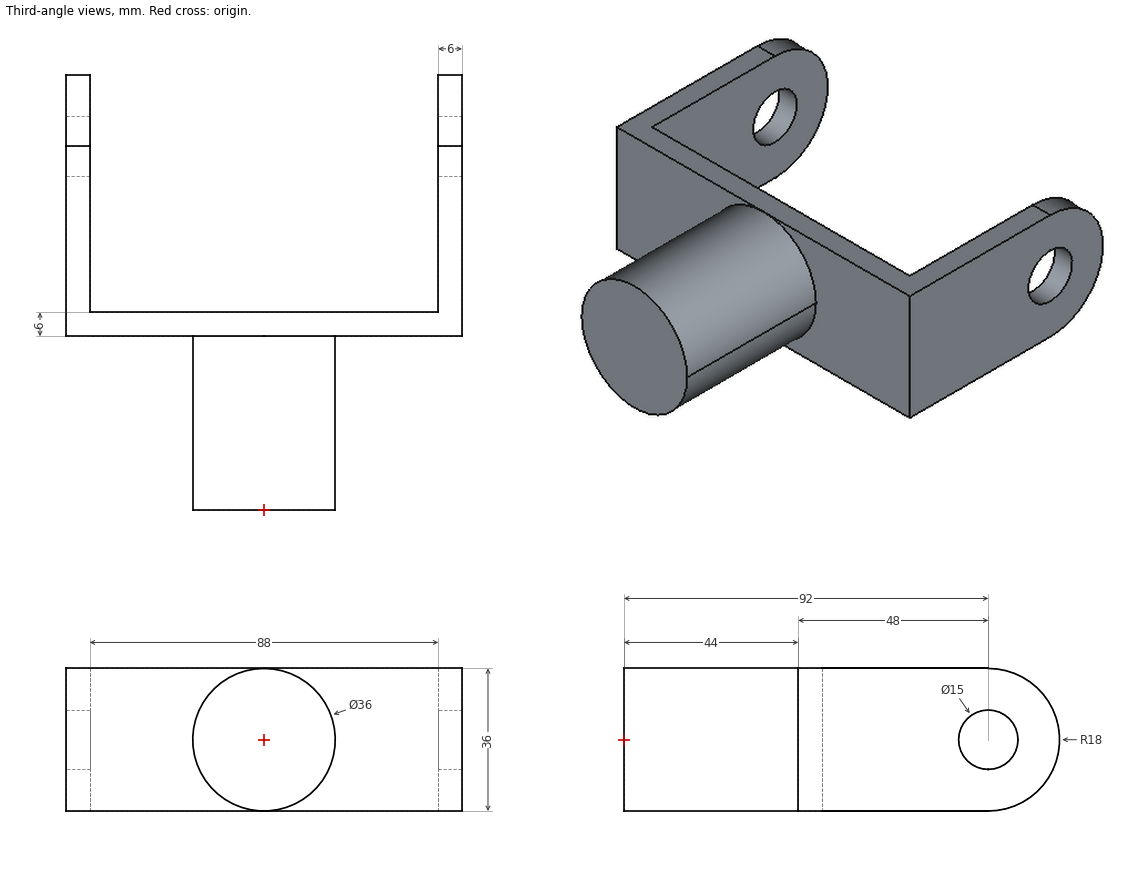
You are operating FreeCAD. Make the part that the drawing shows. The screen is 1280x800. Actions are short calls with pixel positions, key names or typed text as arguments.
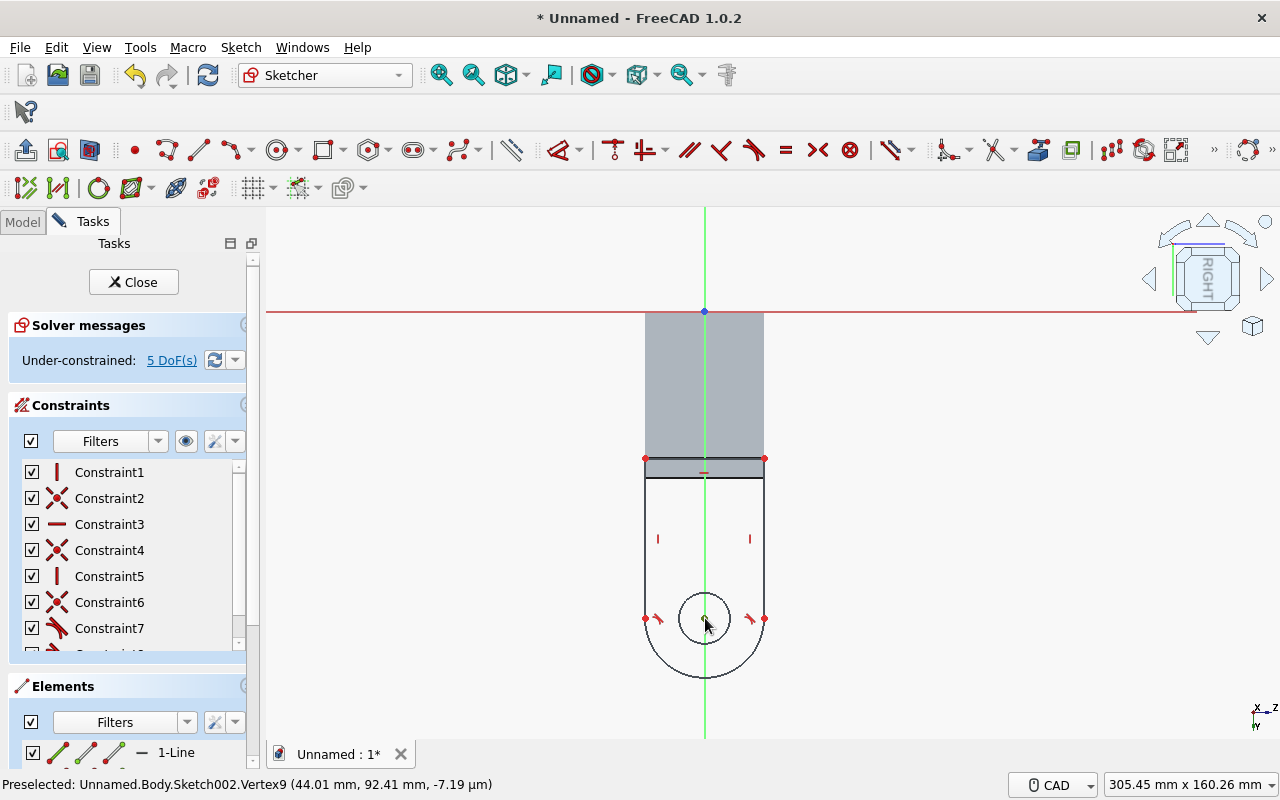
click(705, 541)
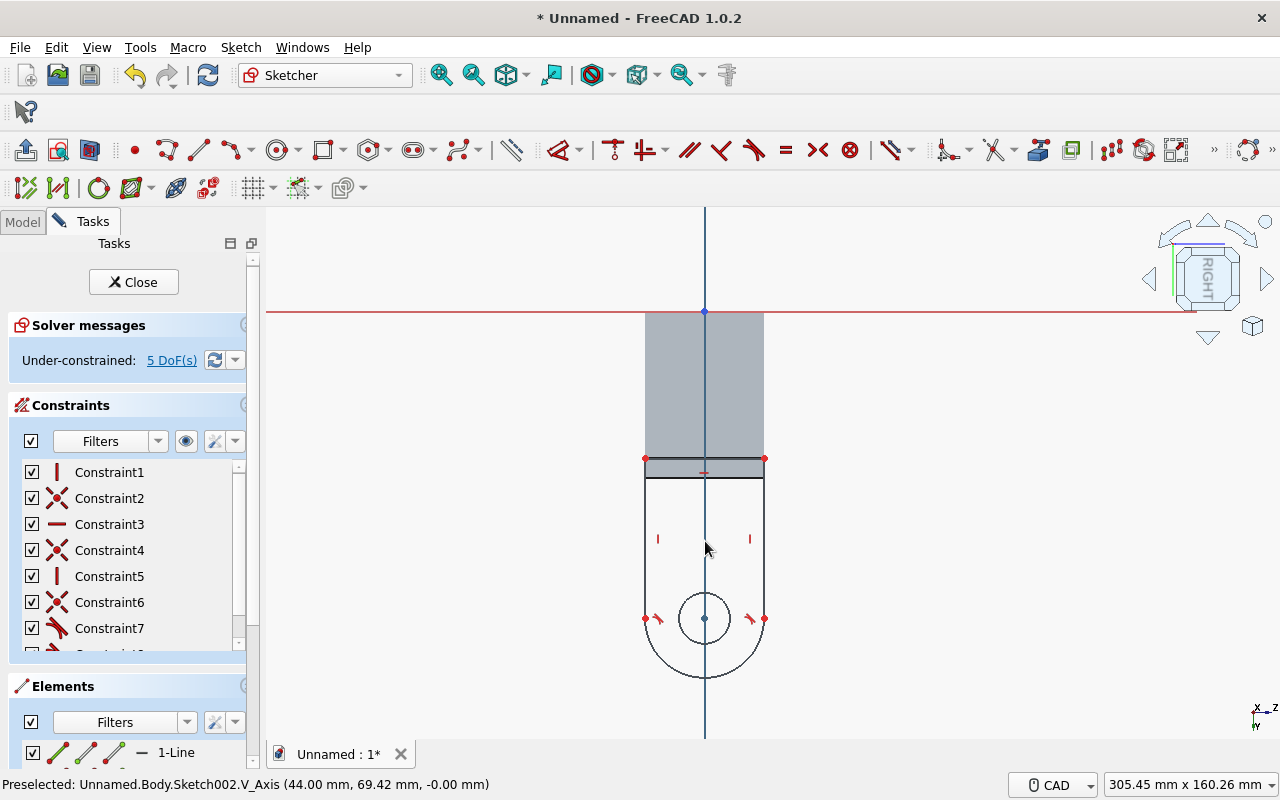
click(614, 150)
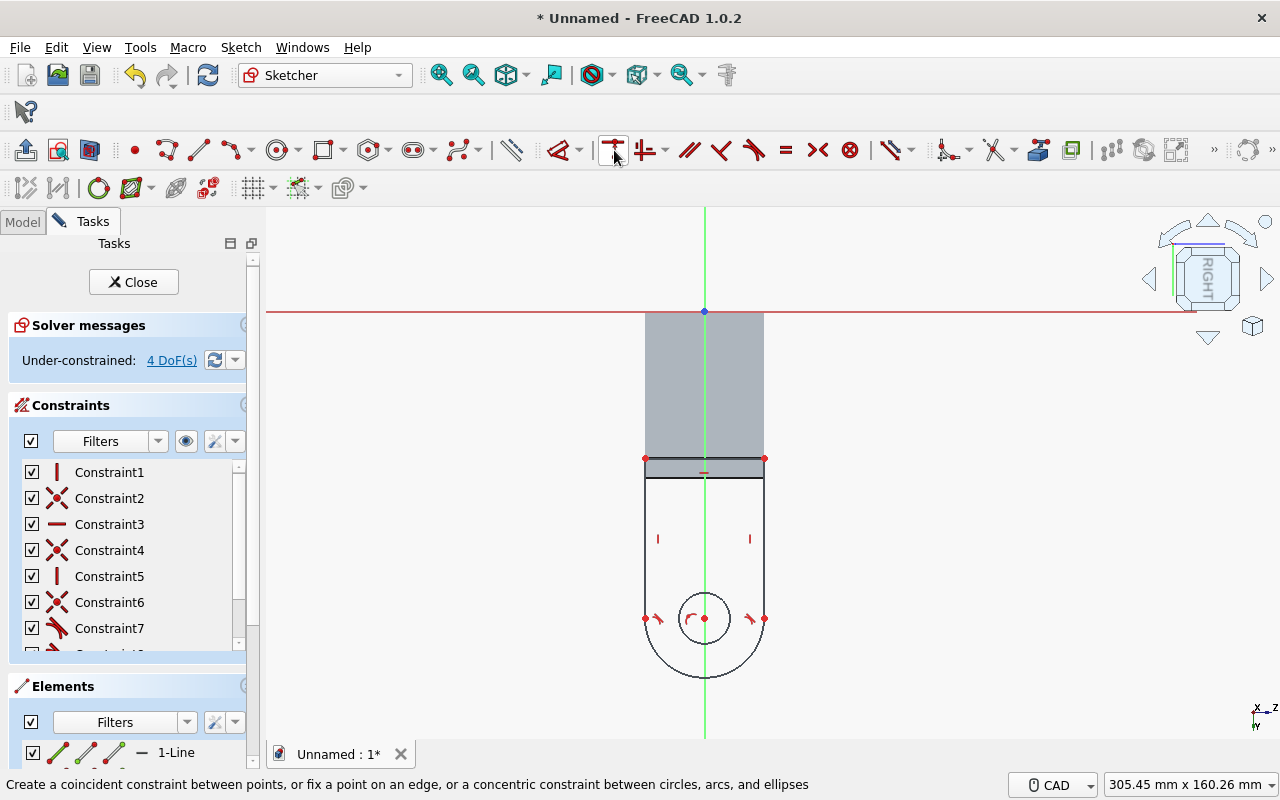
click(670, 666)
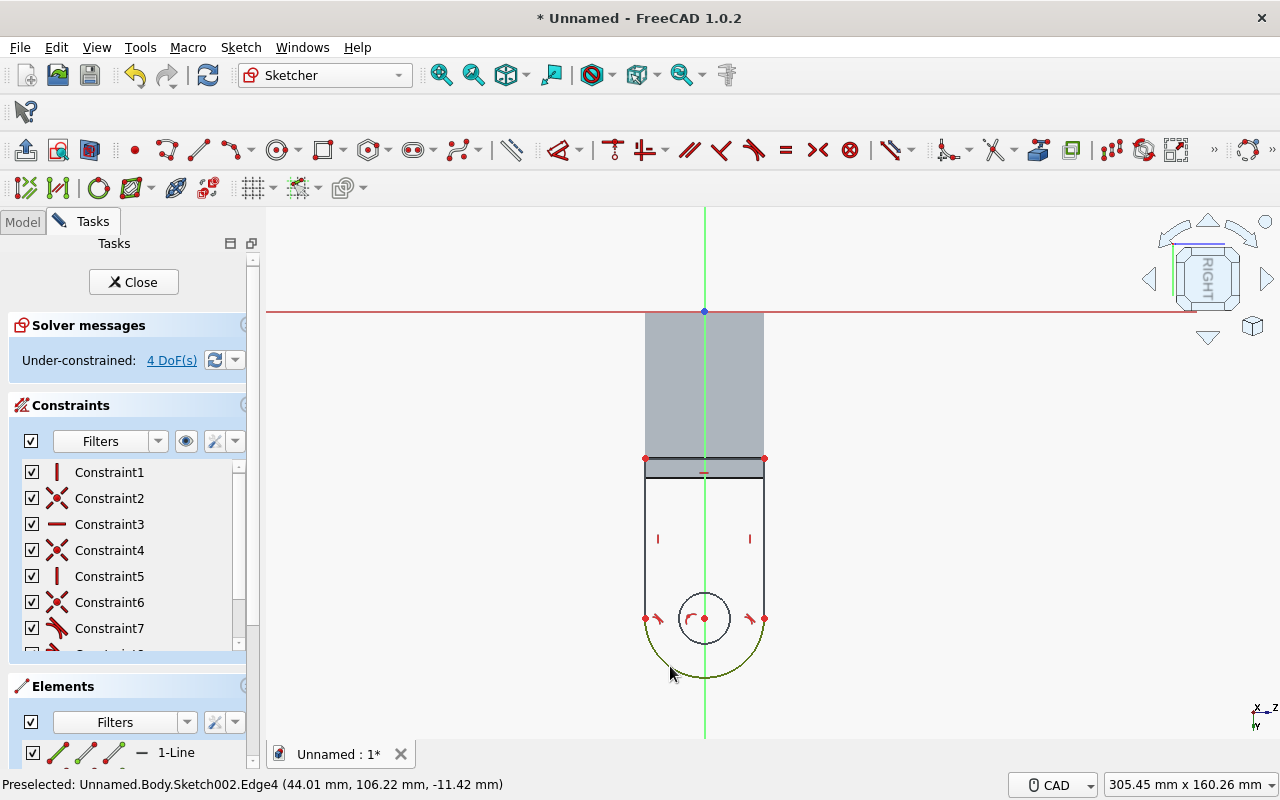
click(582, 150)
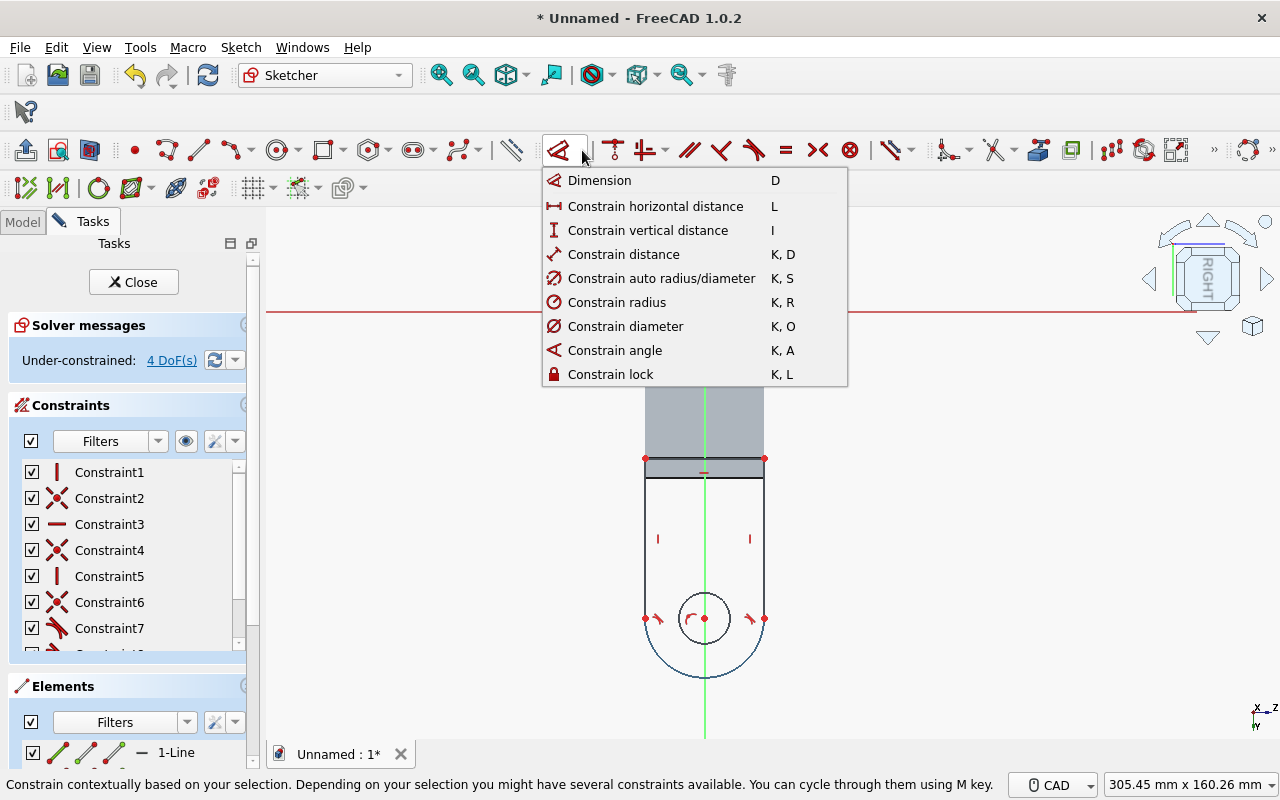
click(695, 302)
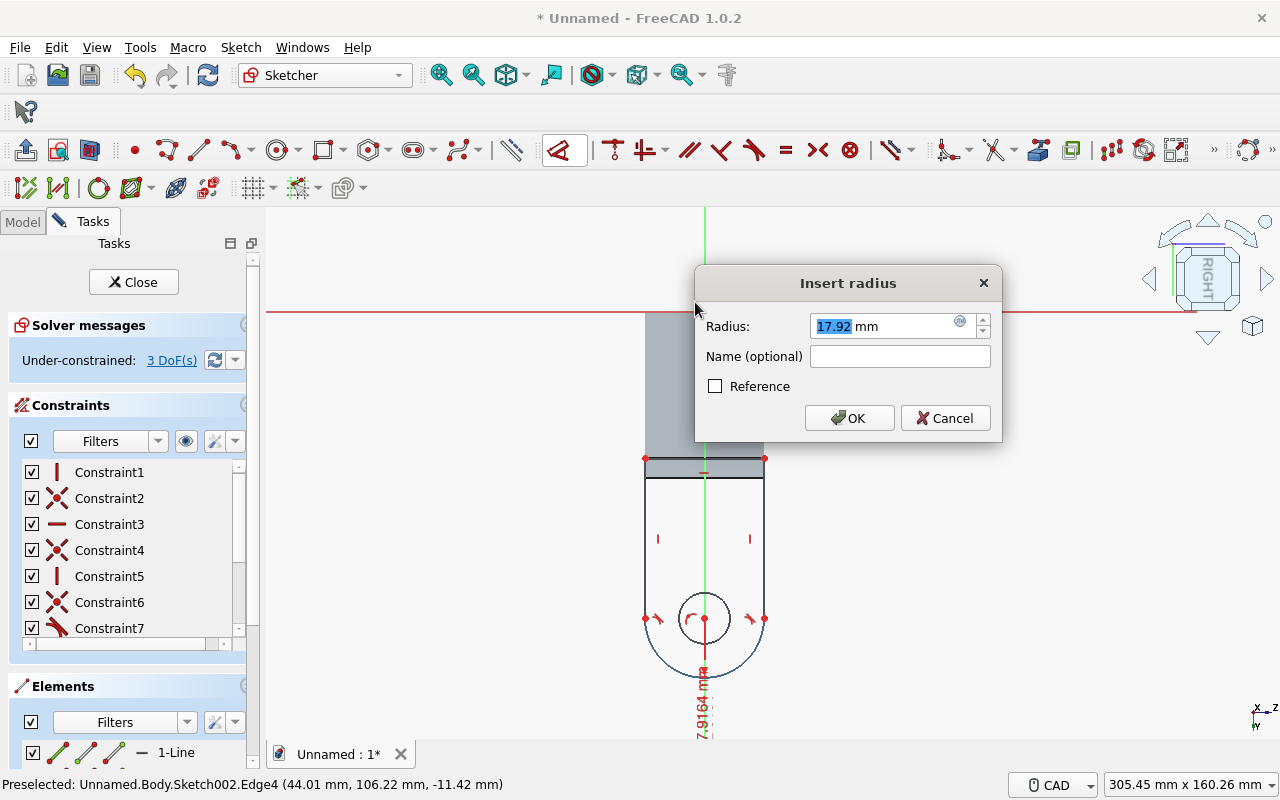
text(18)
key(Return)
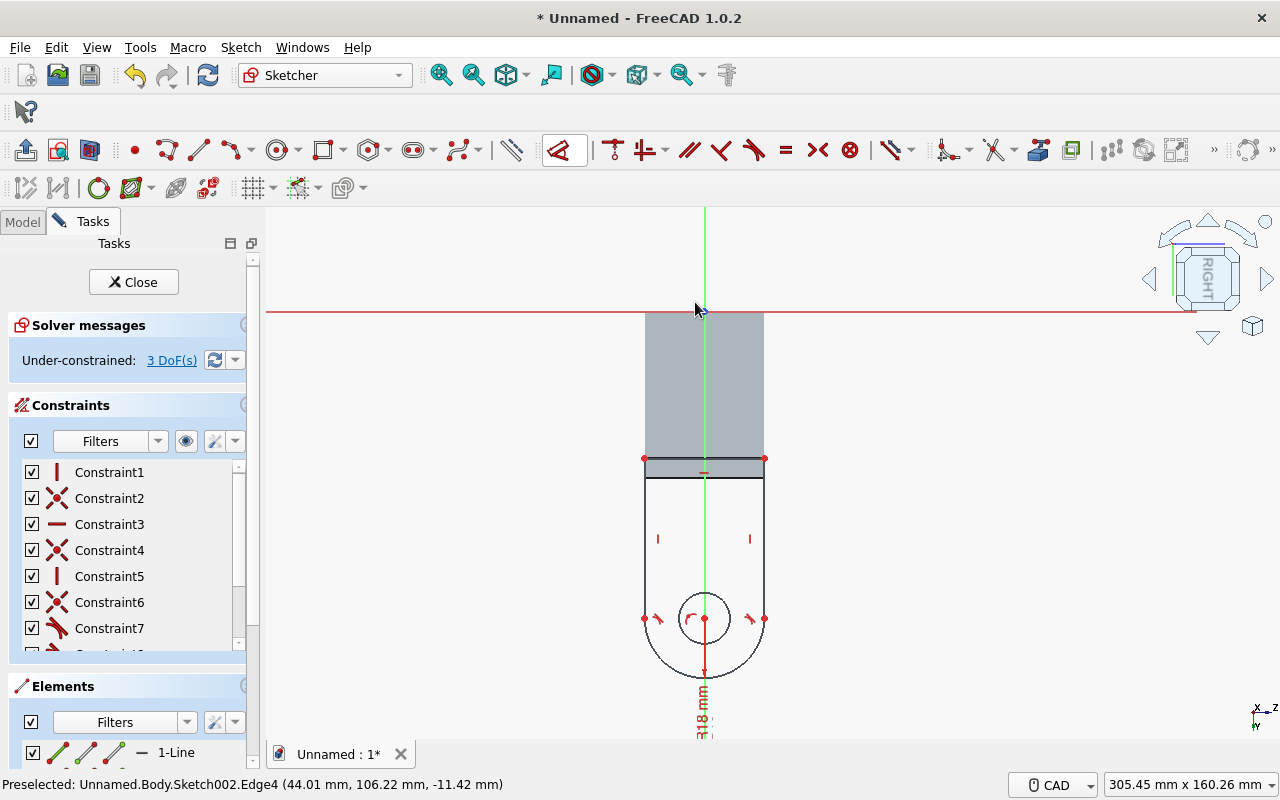
click(722, 600)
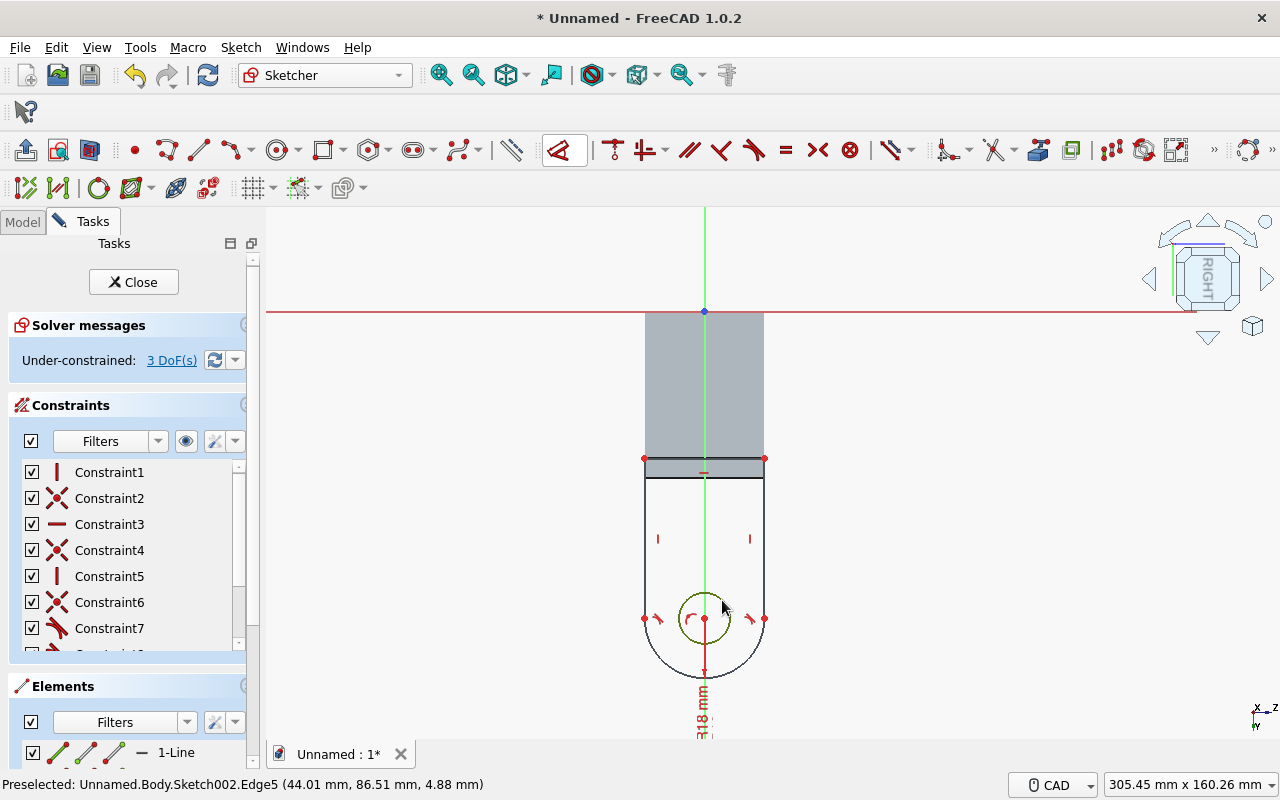
key(k)
key(o)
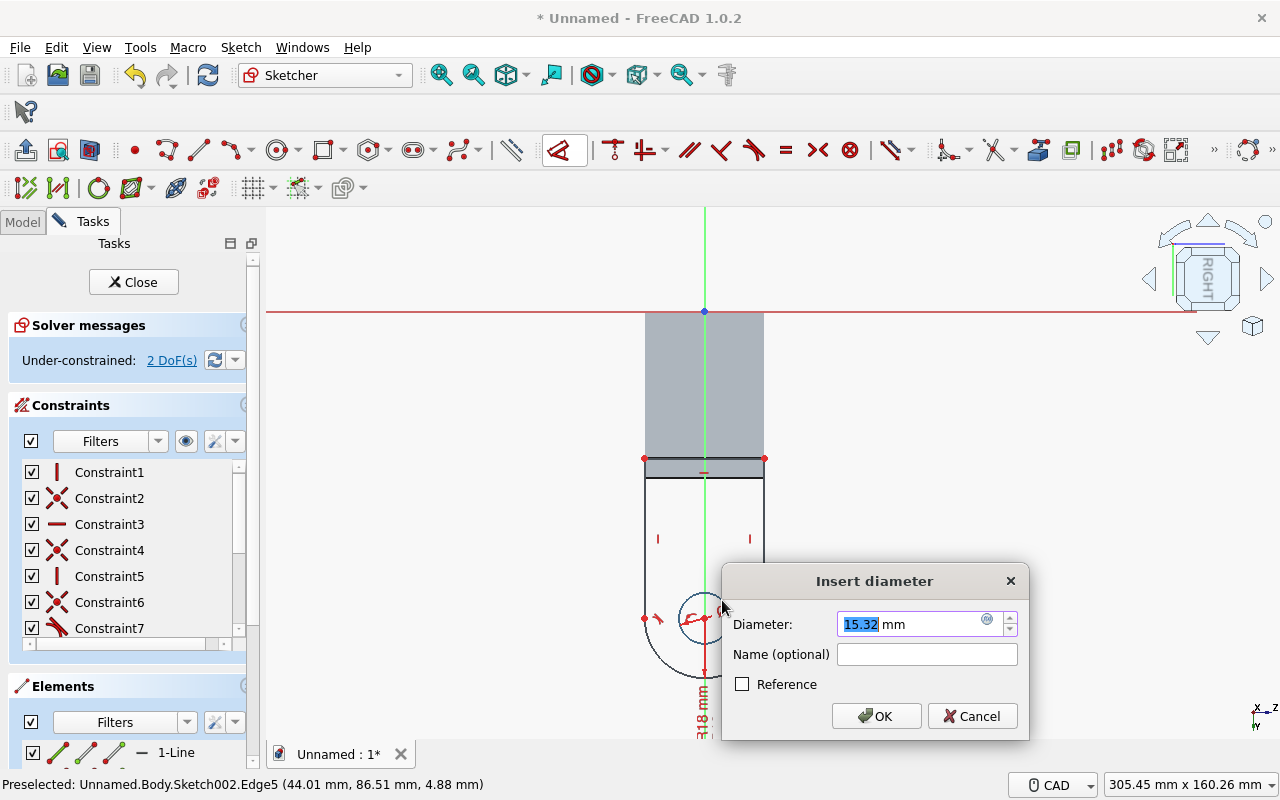
text(15)
key(Return)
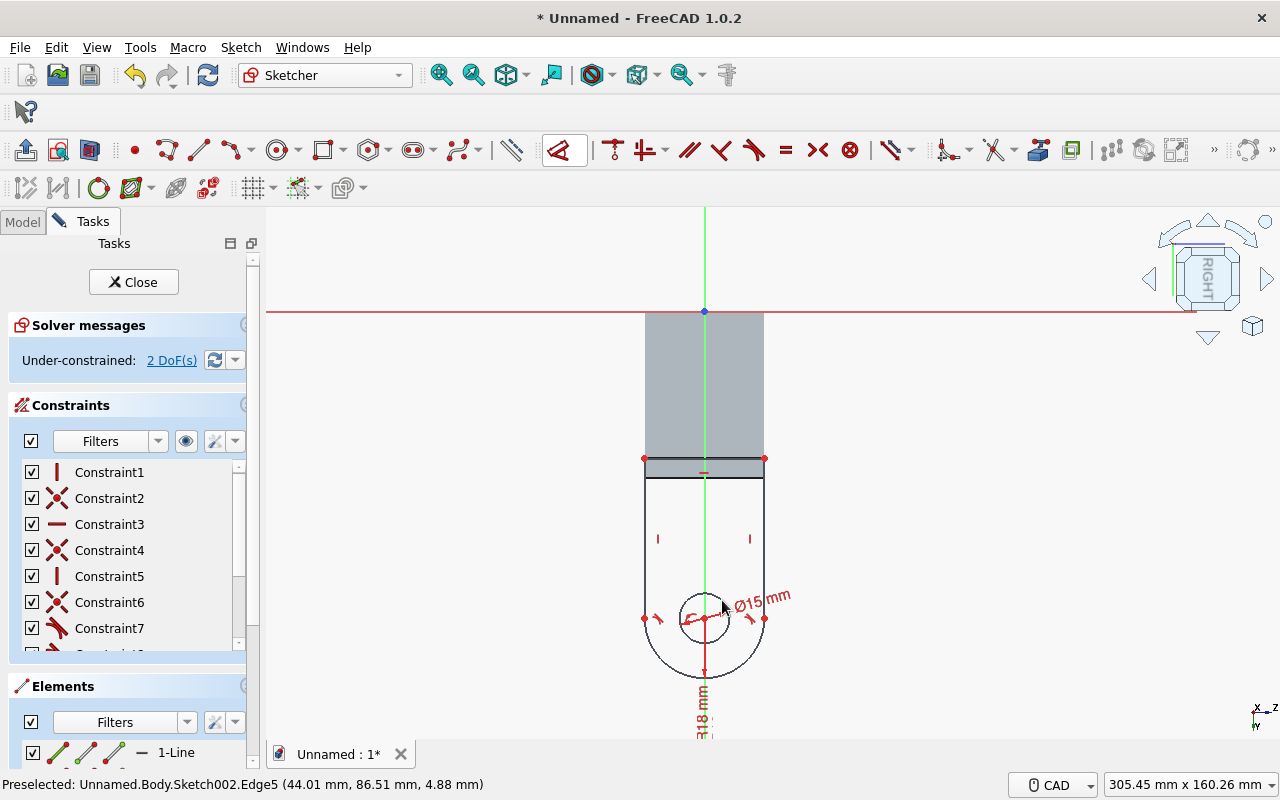
click(764, 571)